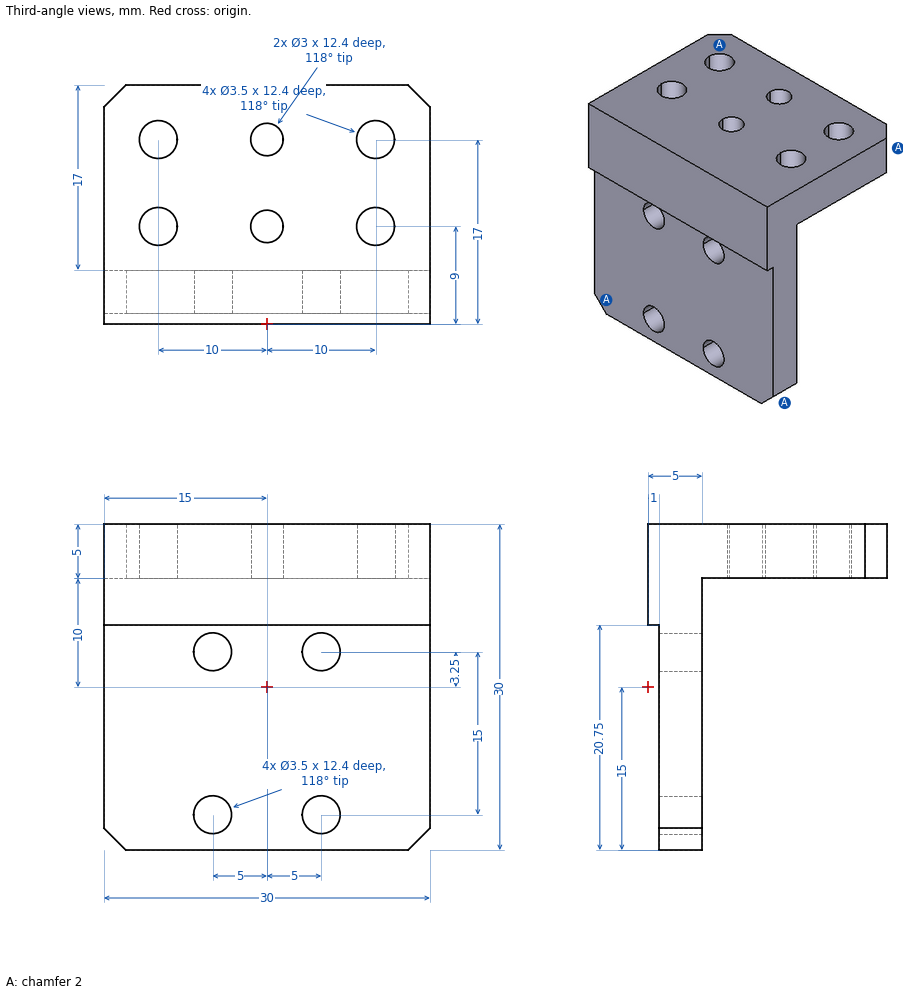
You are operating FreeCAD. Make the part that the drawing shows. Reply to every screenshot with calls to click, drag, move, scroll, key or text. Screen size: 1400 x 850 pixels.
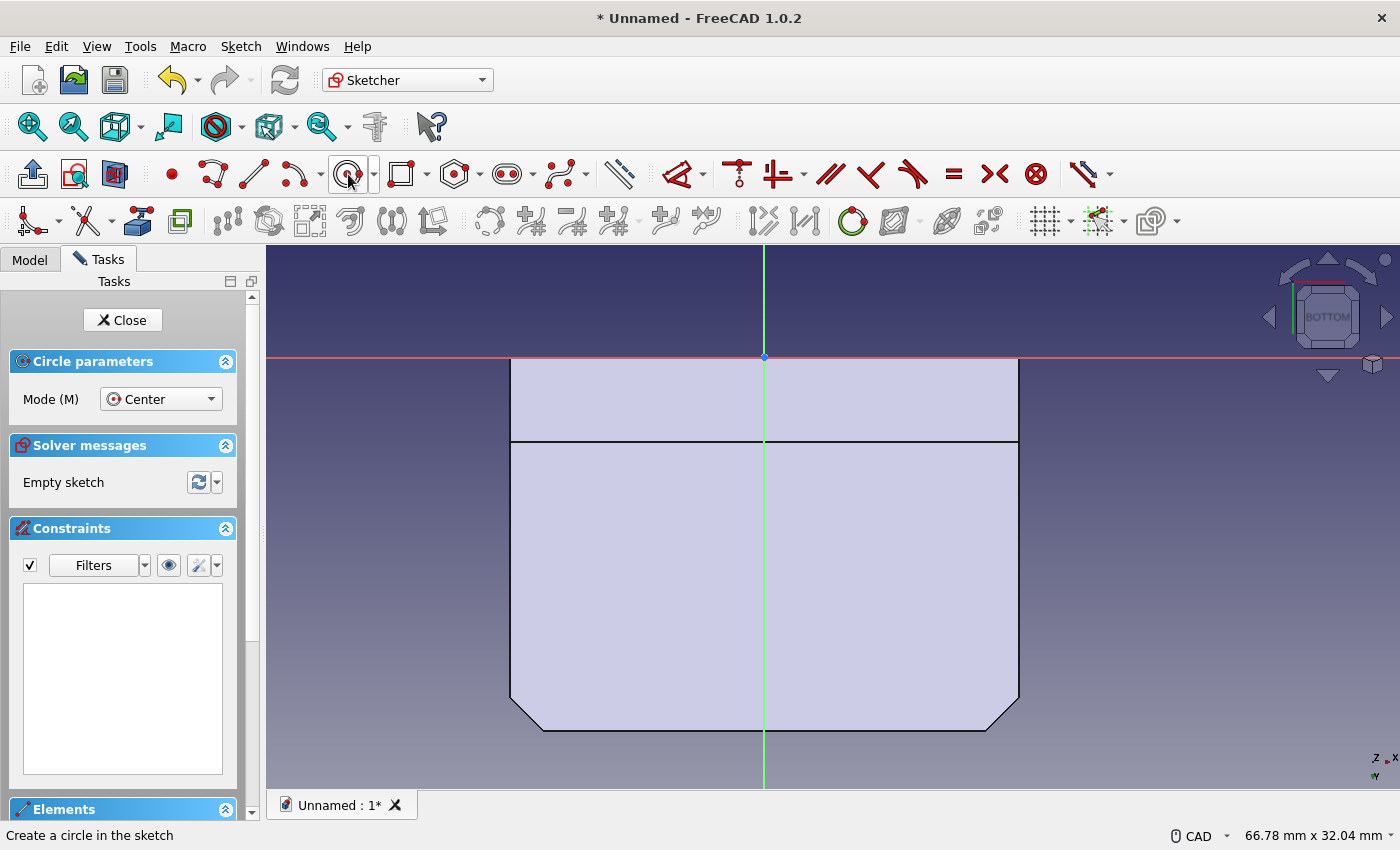
click(934, 646)
click(955, 625)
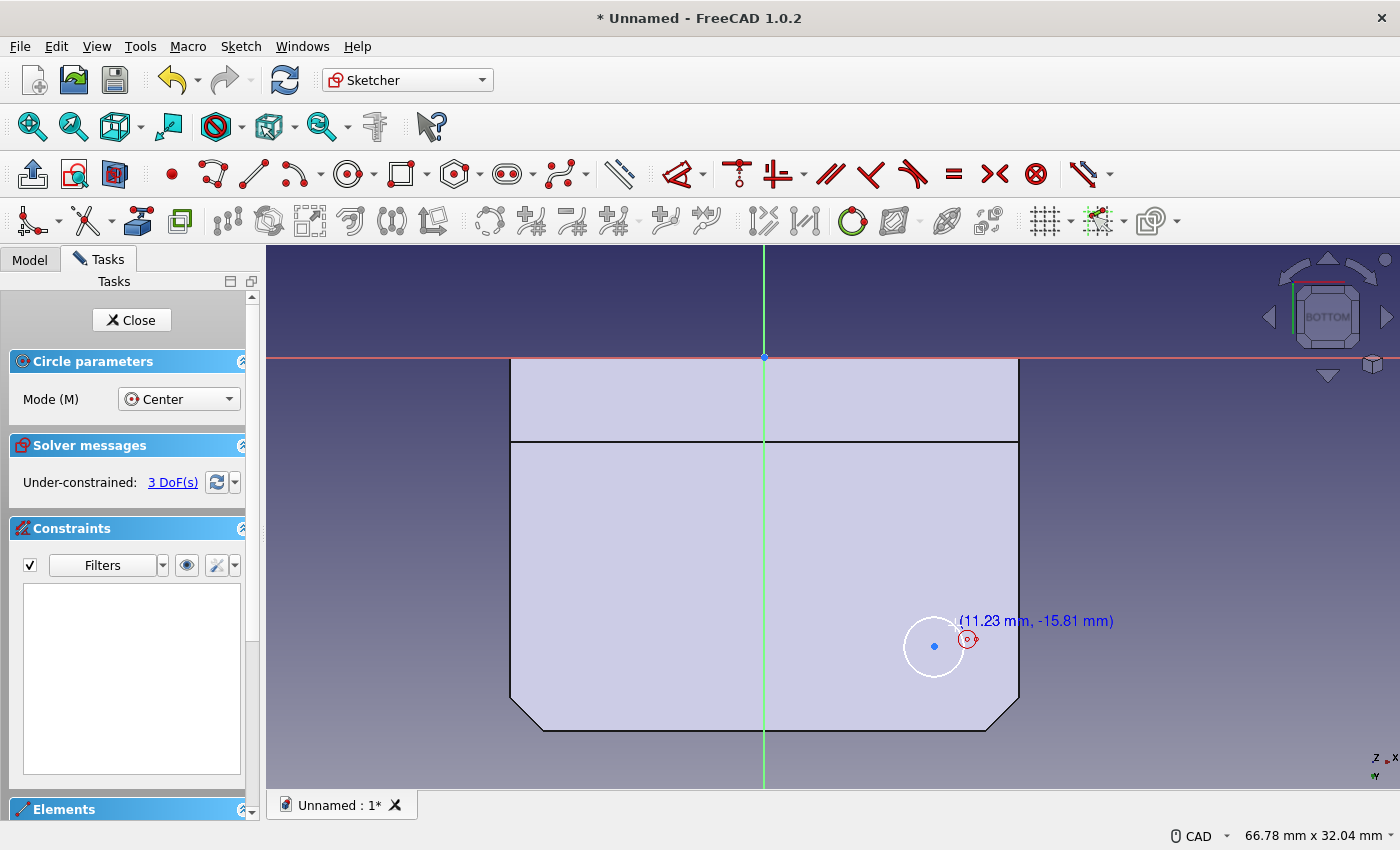
click(595, 646)
click(616, 625)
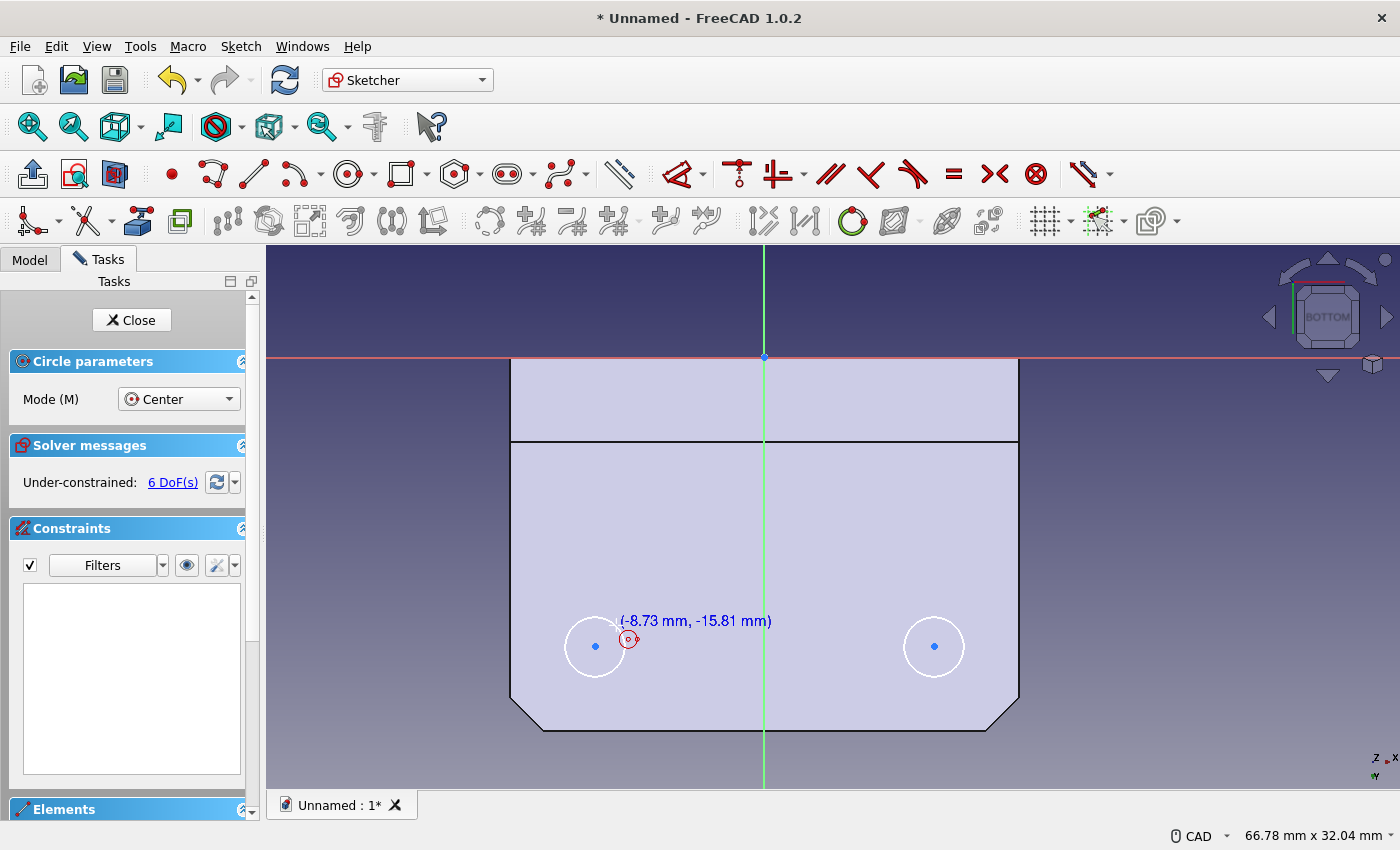
click(934, 510)
click(955, 489)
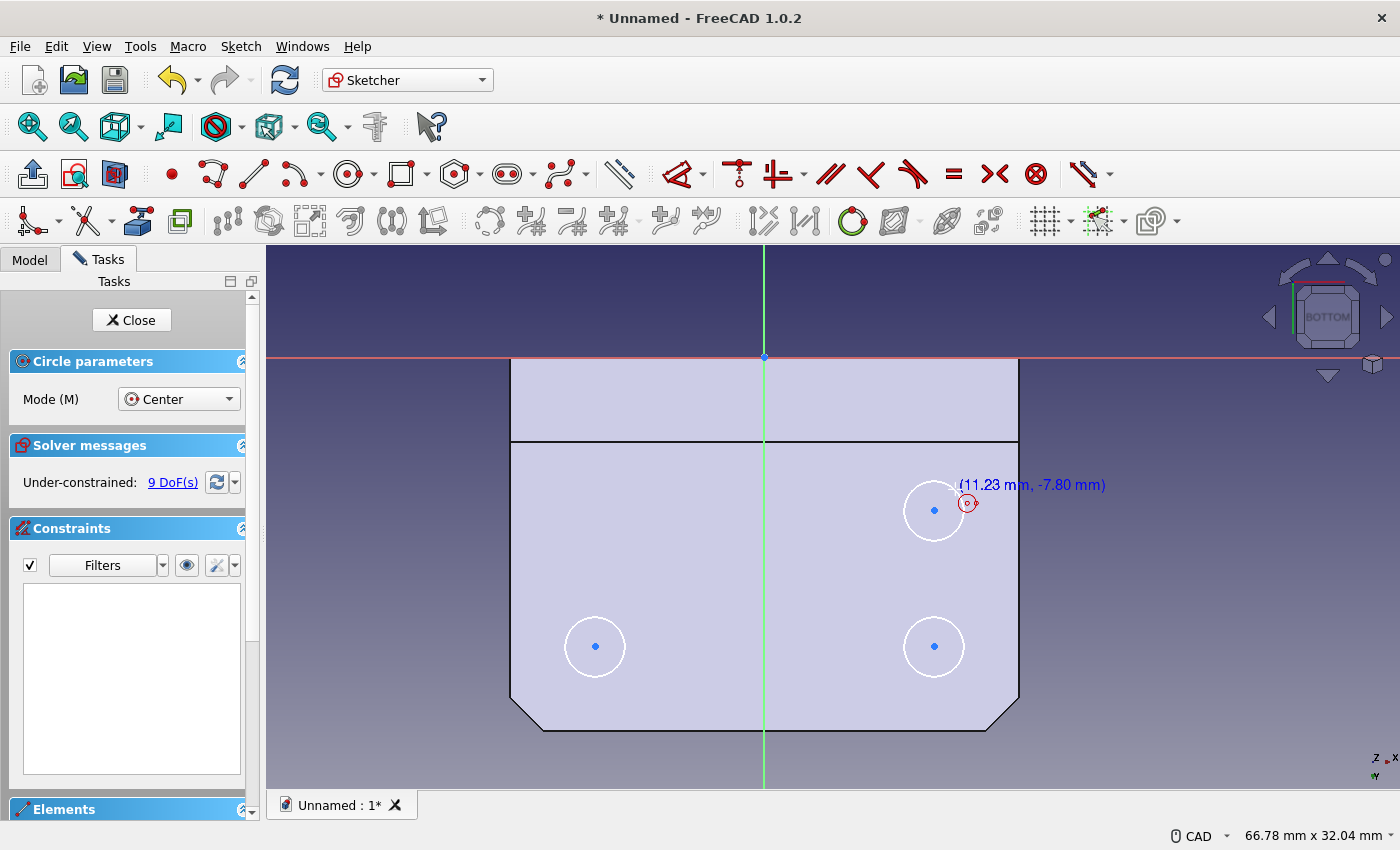
click(595, 510)
click(616, 489)
key(Escape)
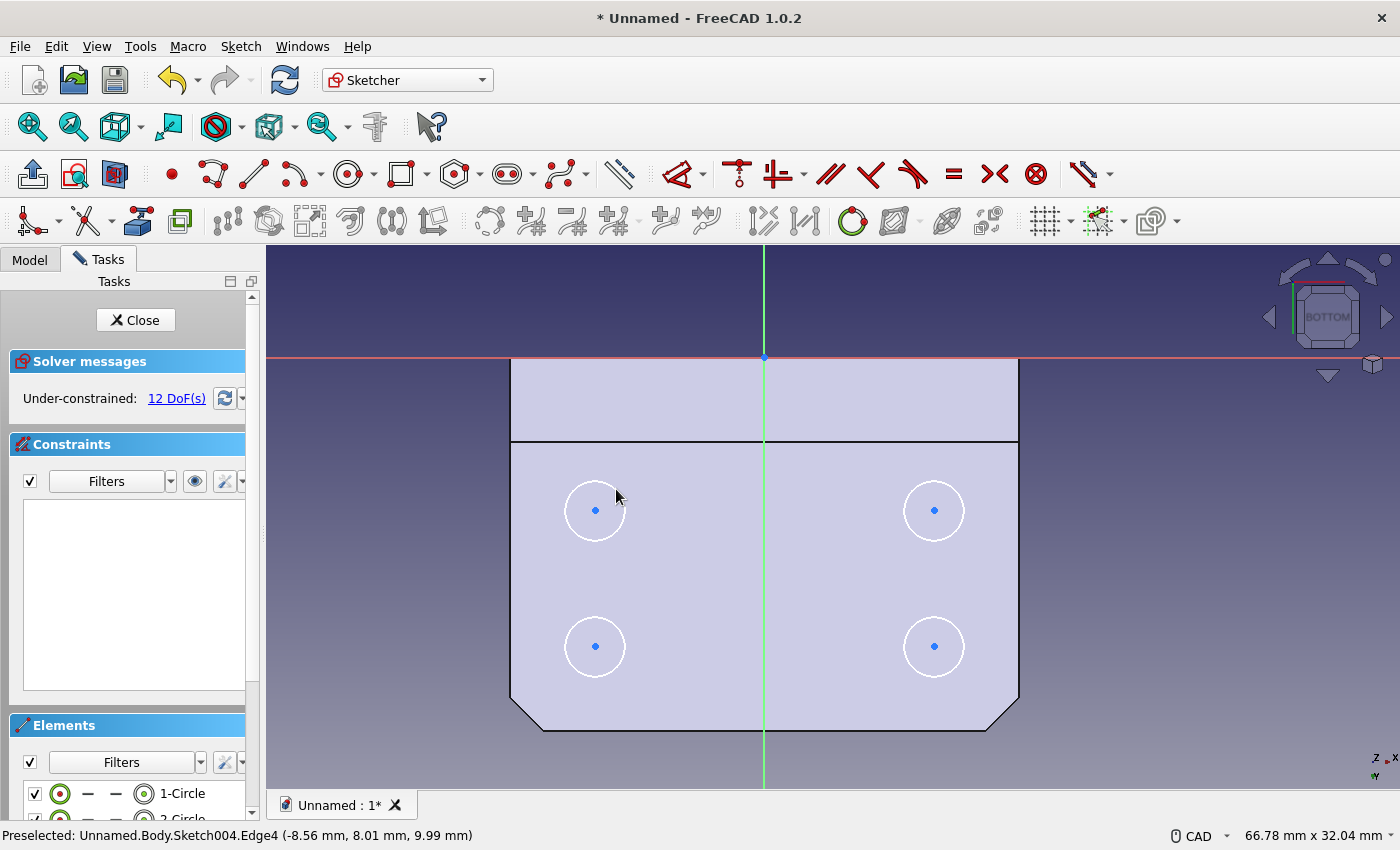
click(955, 626)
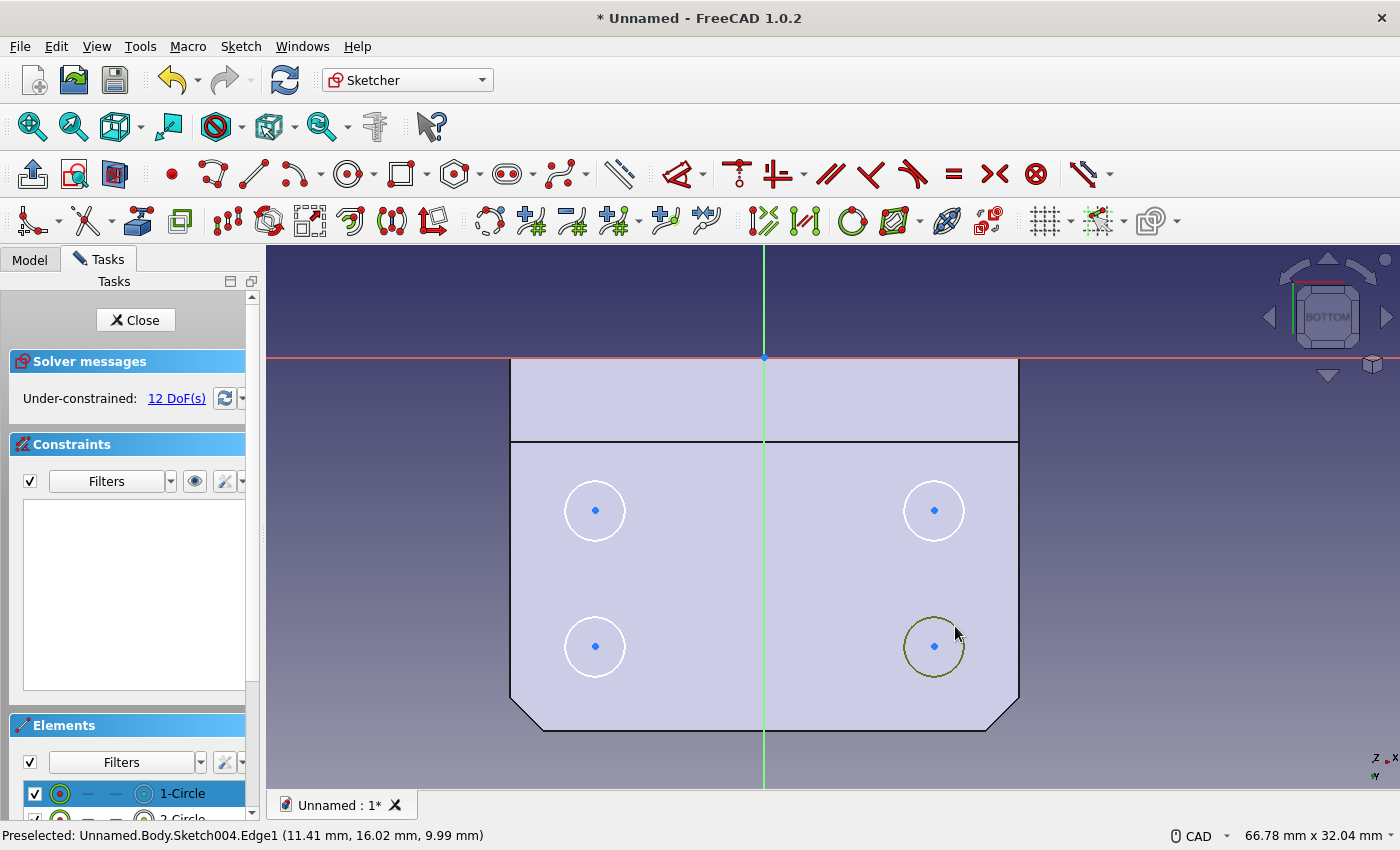
click(616, 626)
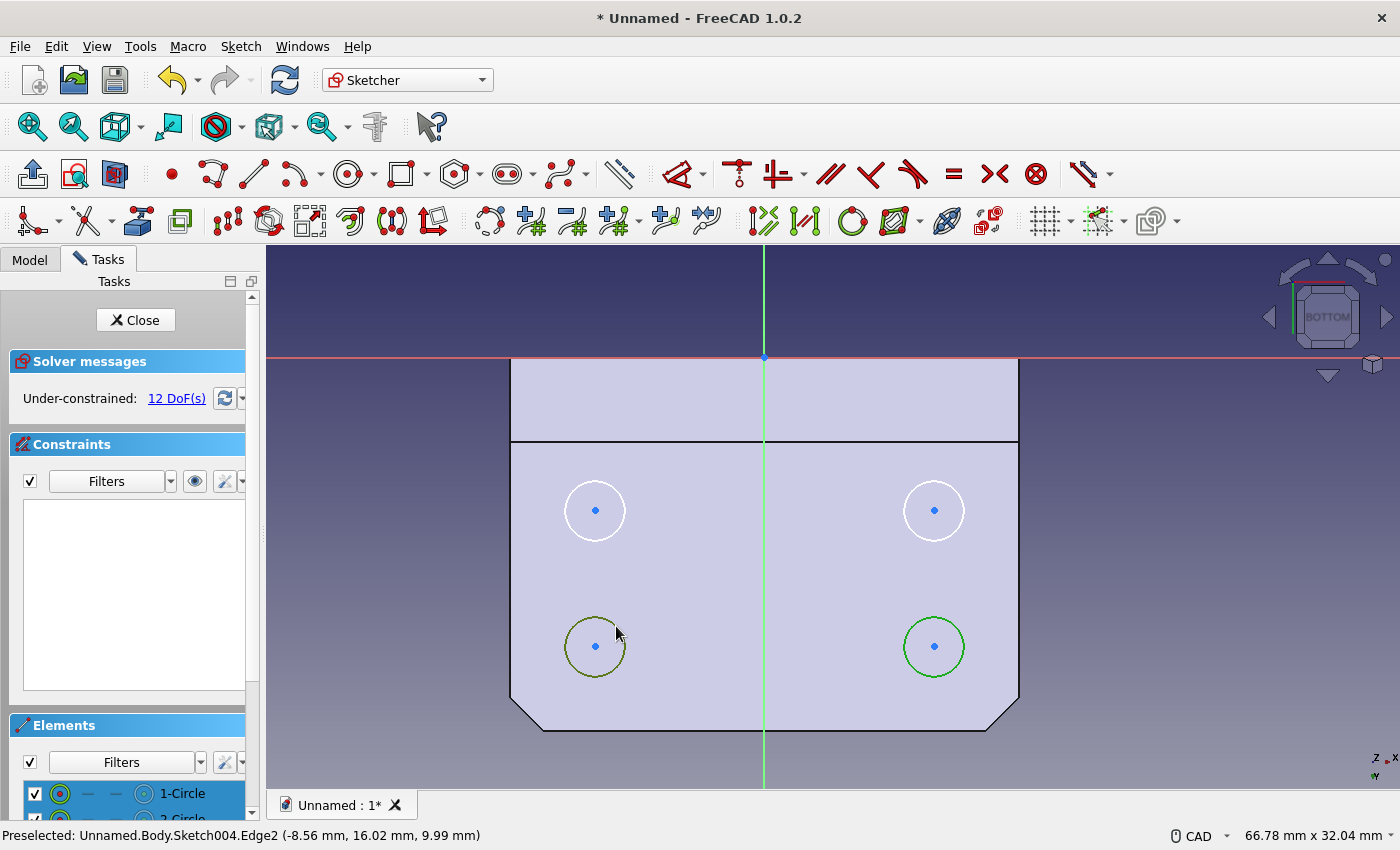
click(955, 490)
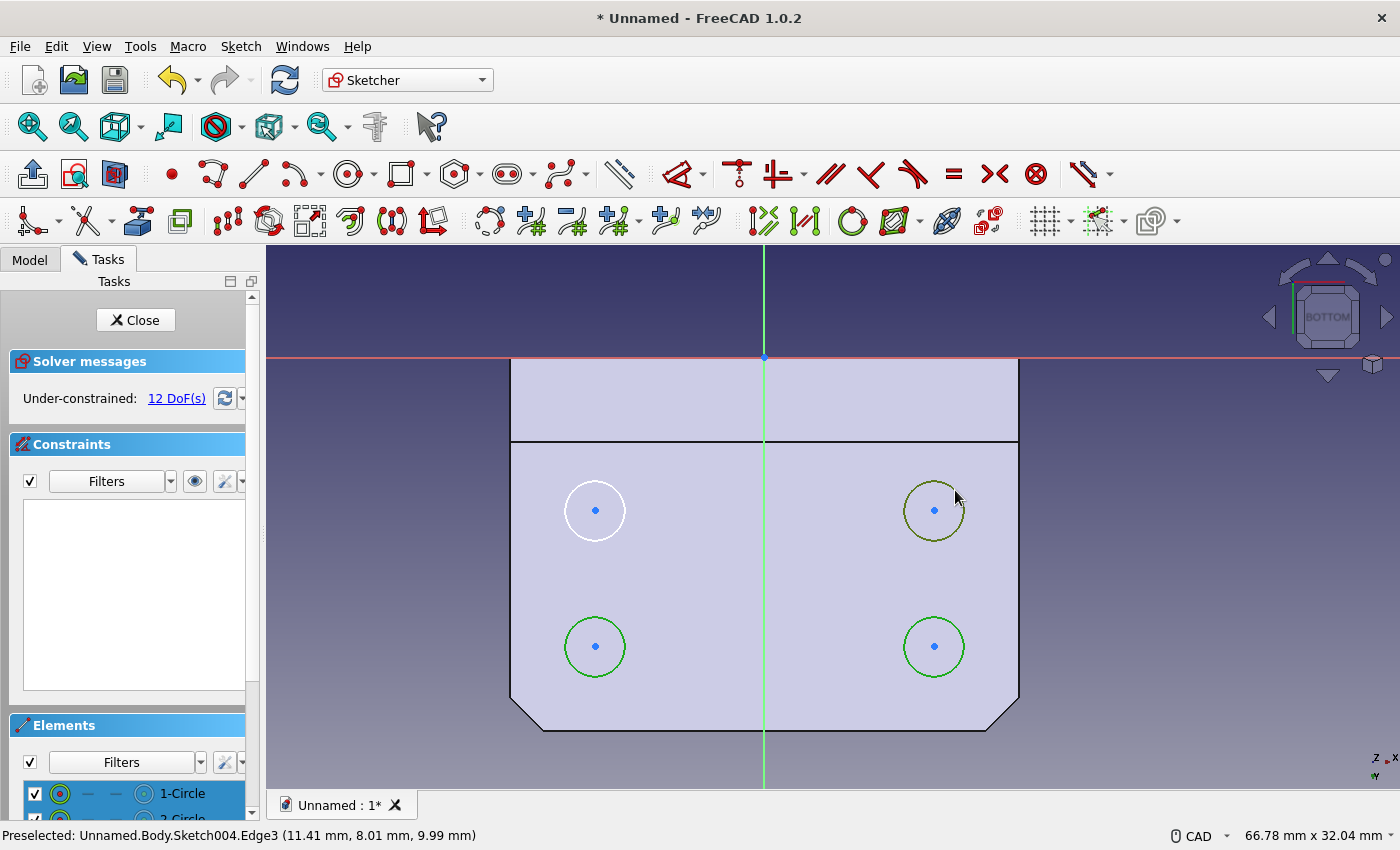
click(616, 490)